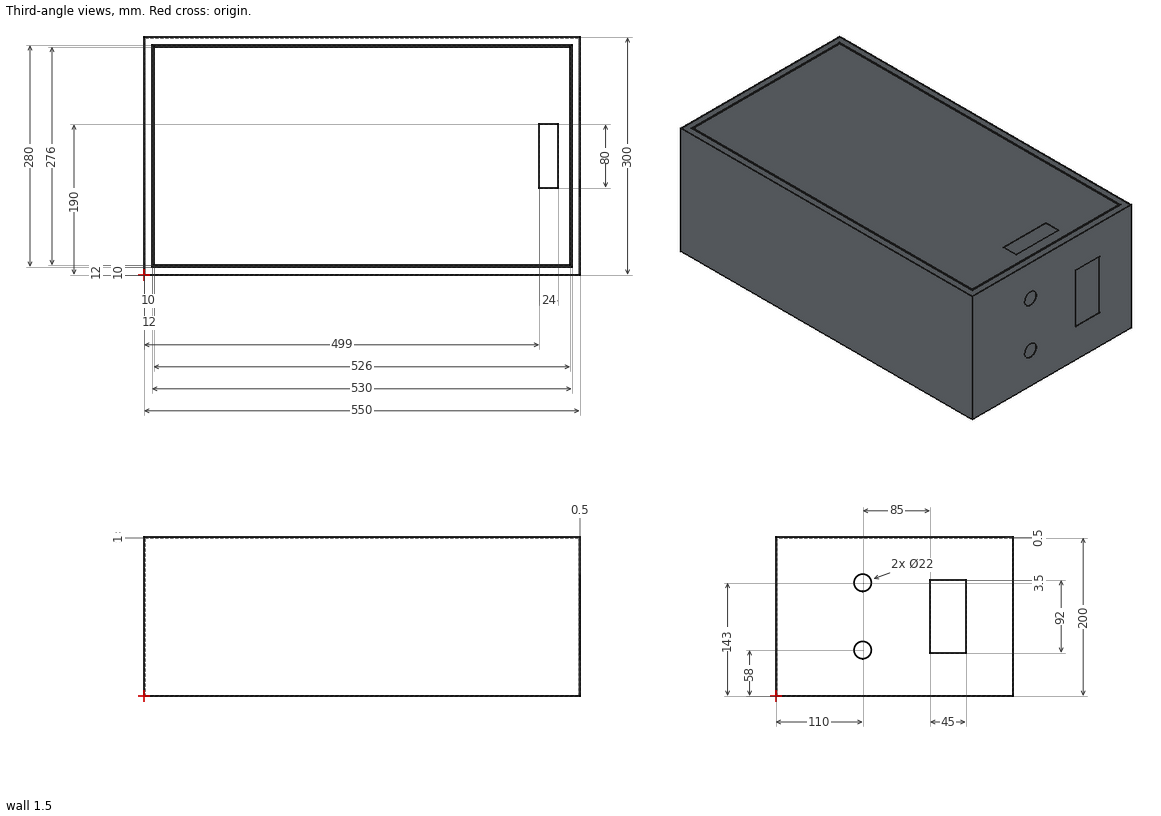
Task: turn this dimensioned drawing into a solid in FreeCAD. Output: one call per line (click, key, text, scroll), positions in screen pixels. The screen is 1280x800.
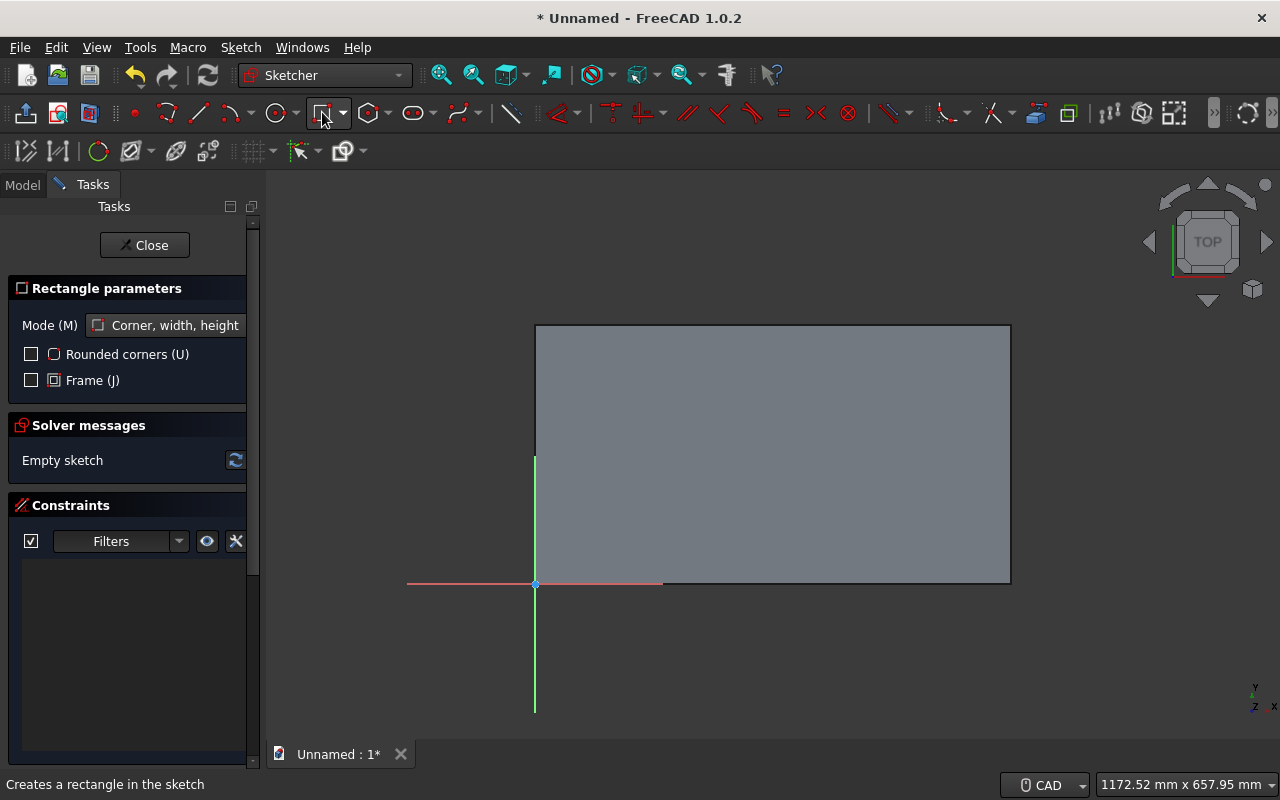
scroll(544, 333, up, 4)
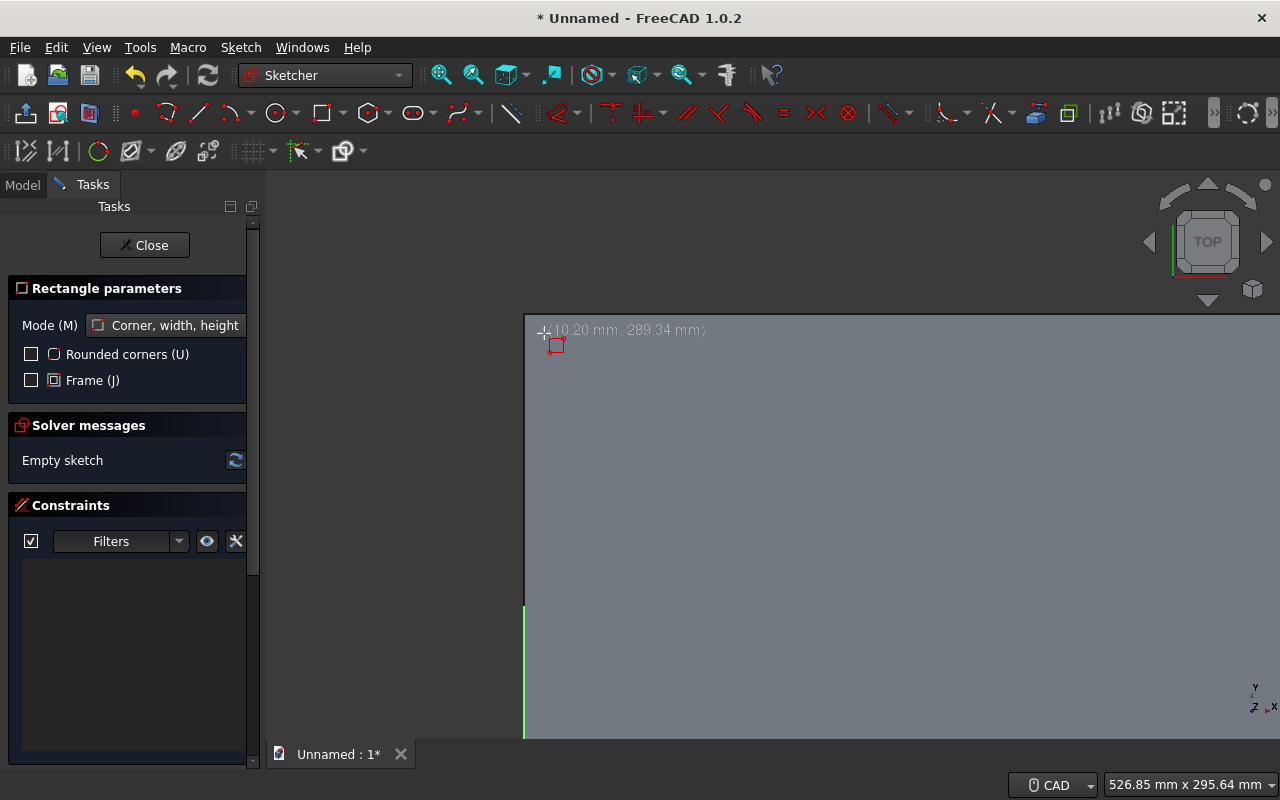
click(543, 334)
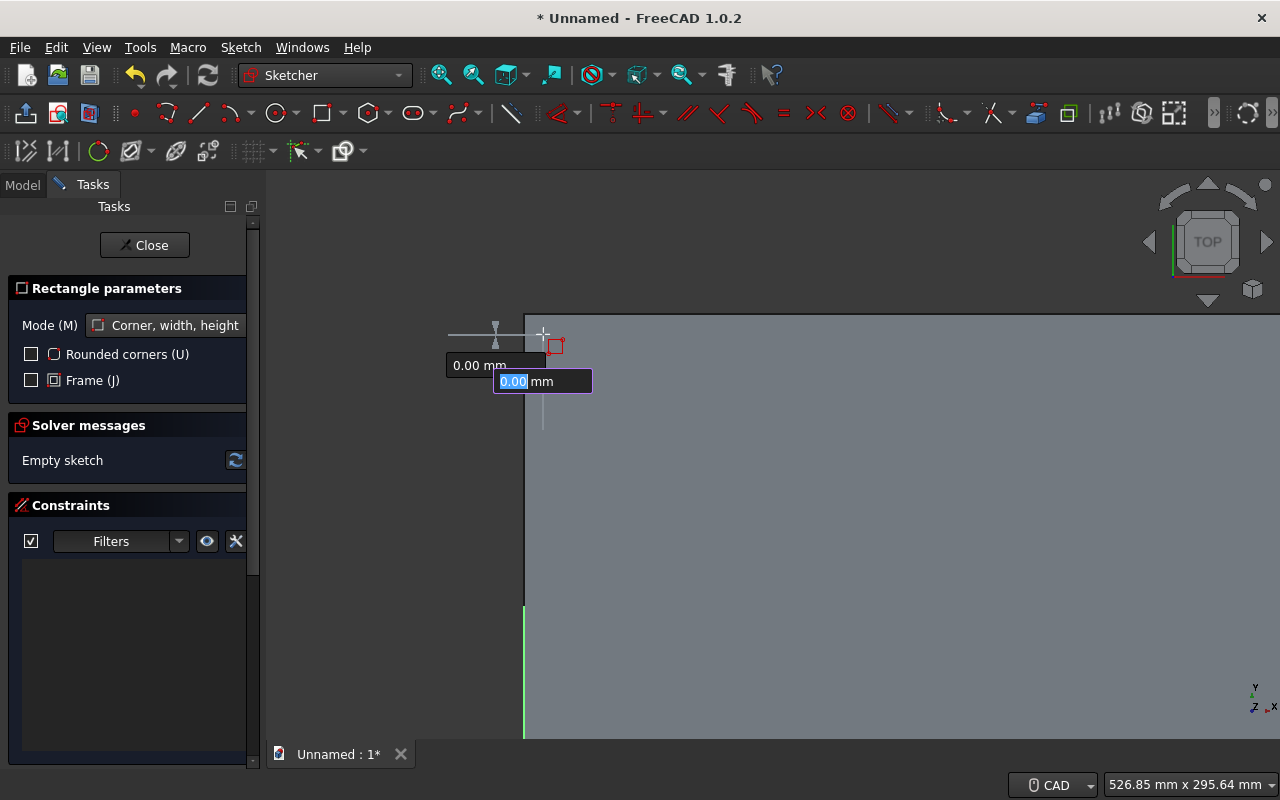
scroll(294, 262, down, 3)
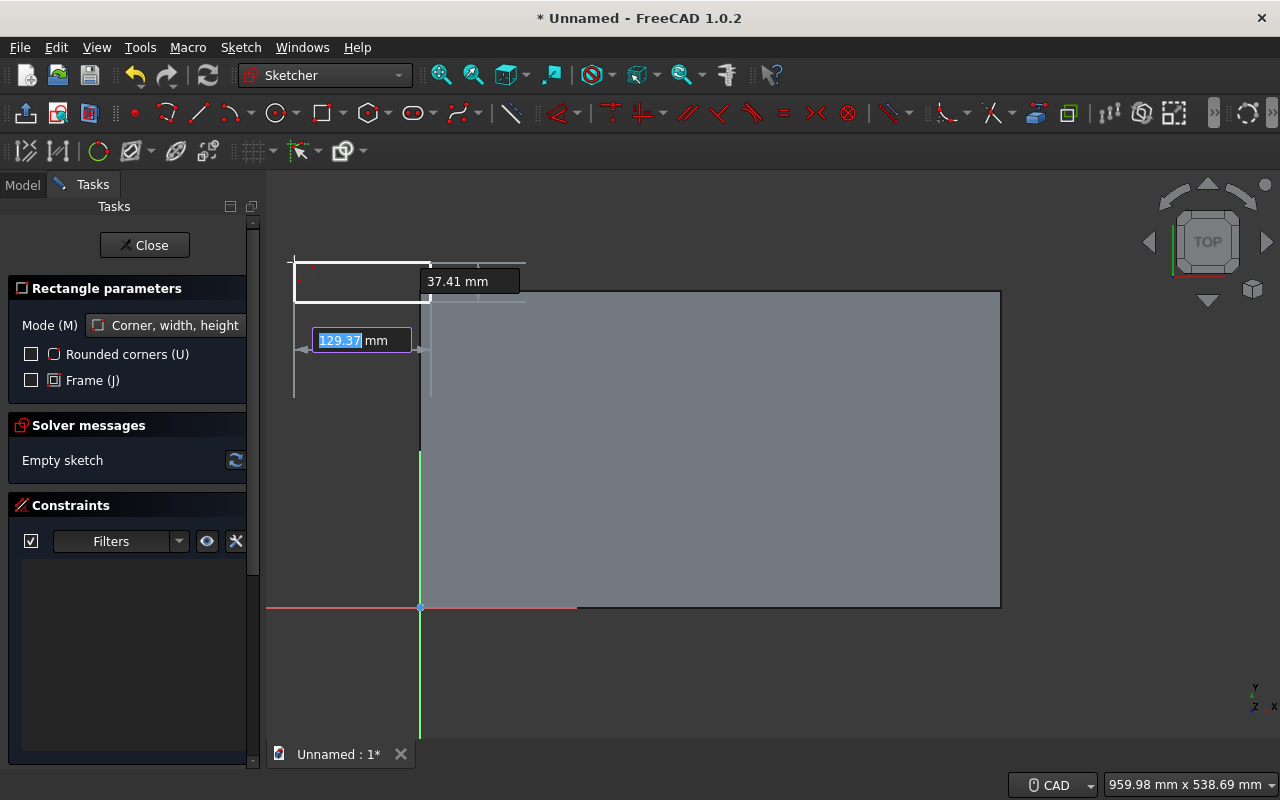
scroll(991, 597, up, 3)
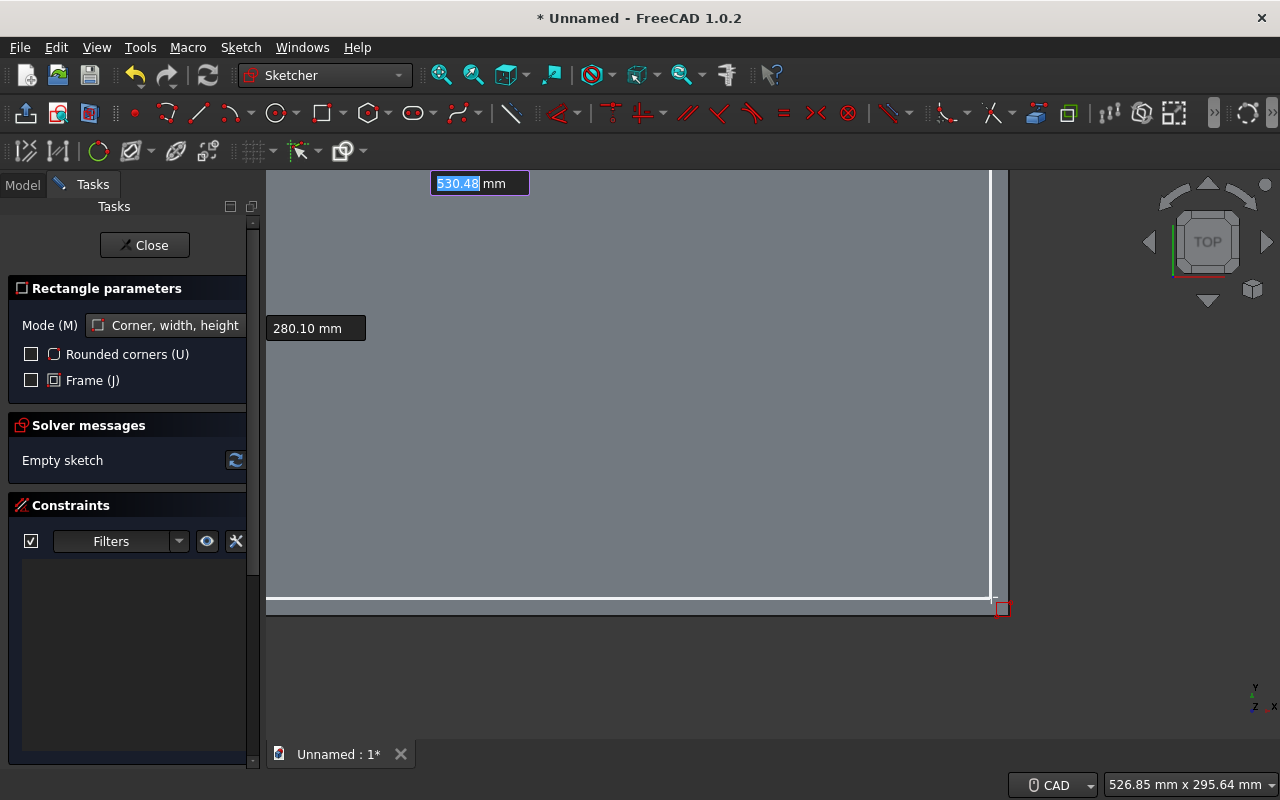
click(990, 597)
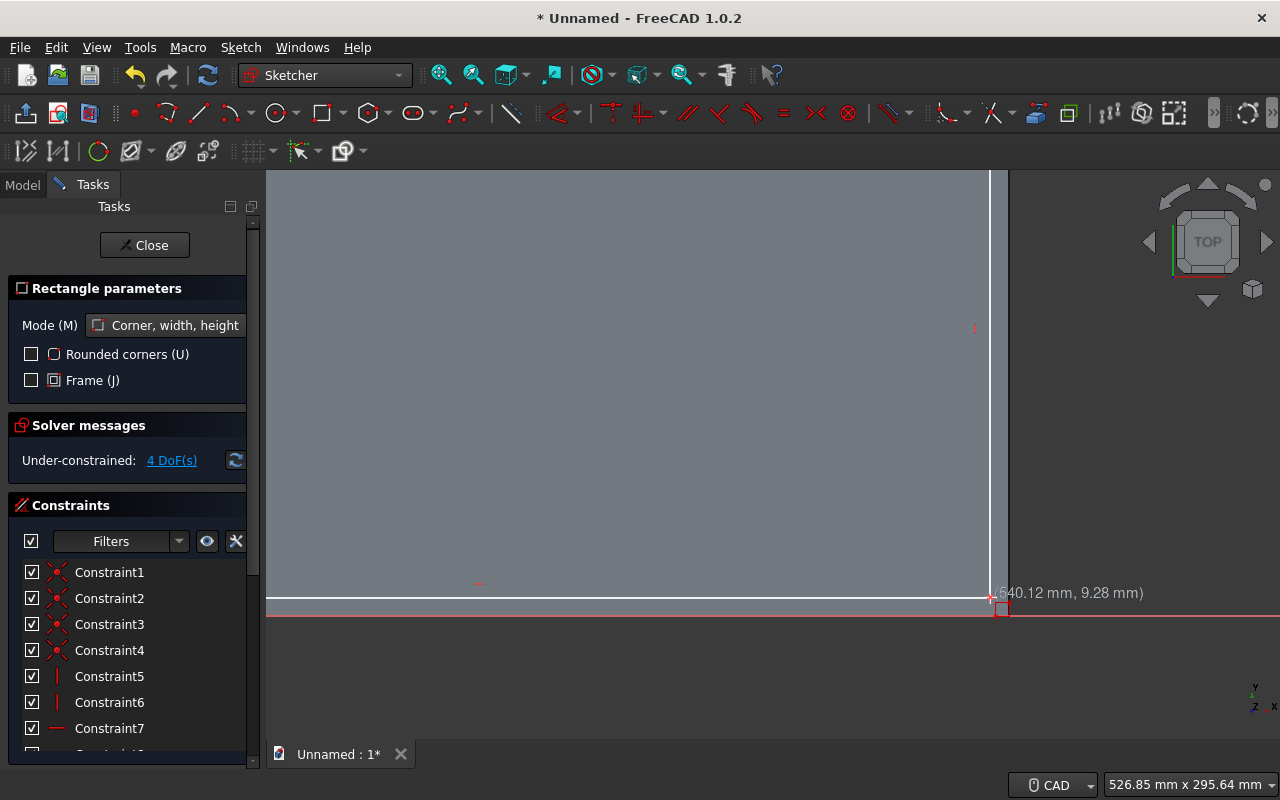
click(911, 250)
move(957, 404)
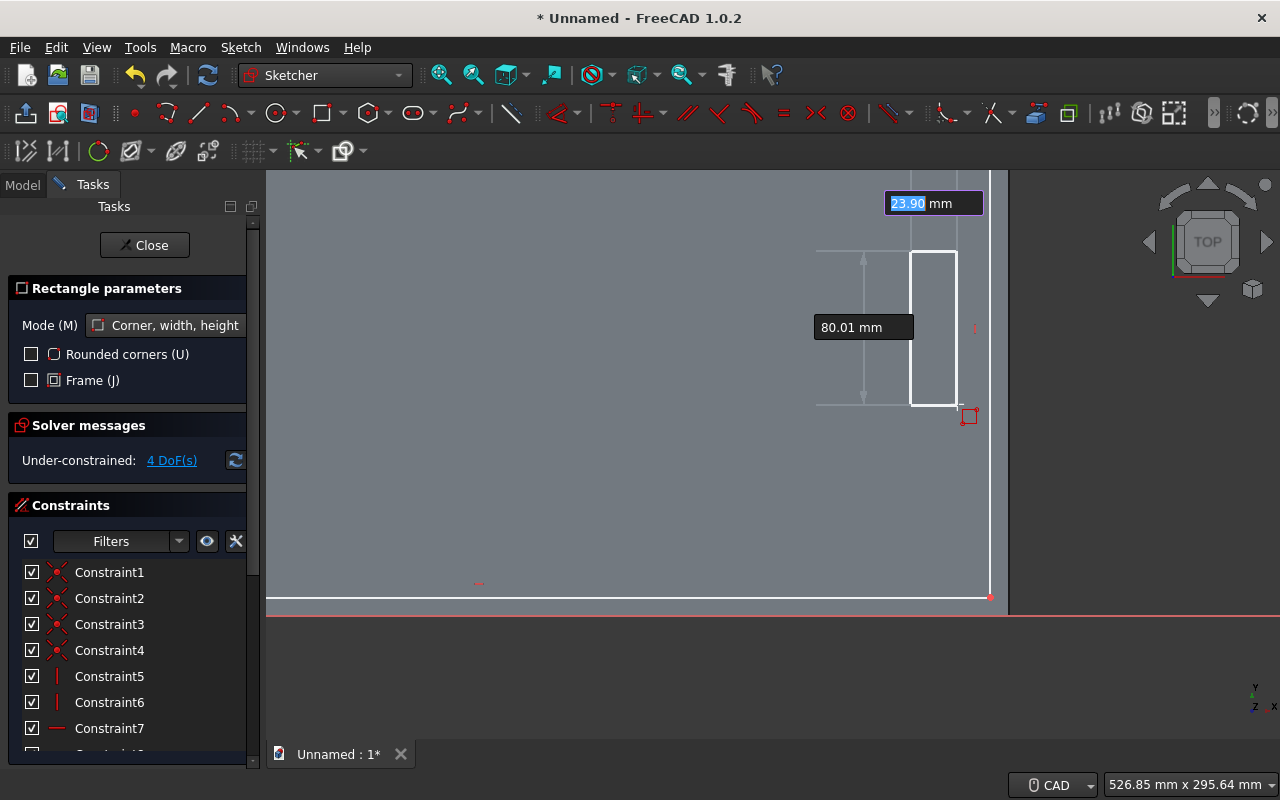
text(24)
key(Tab)
text(80)
key(Return)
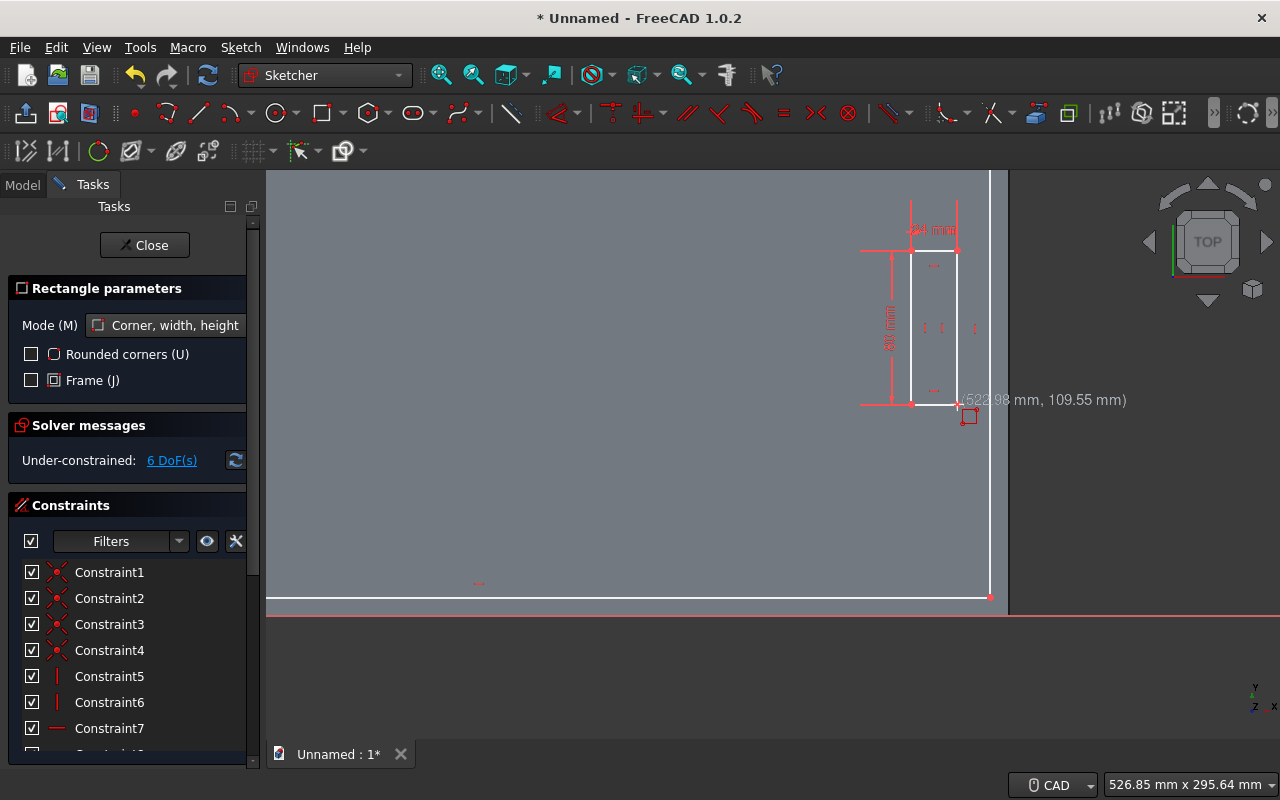
scroll(990, 598, down, 3)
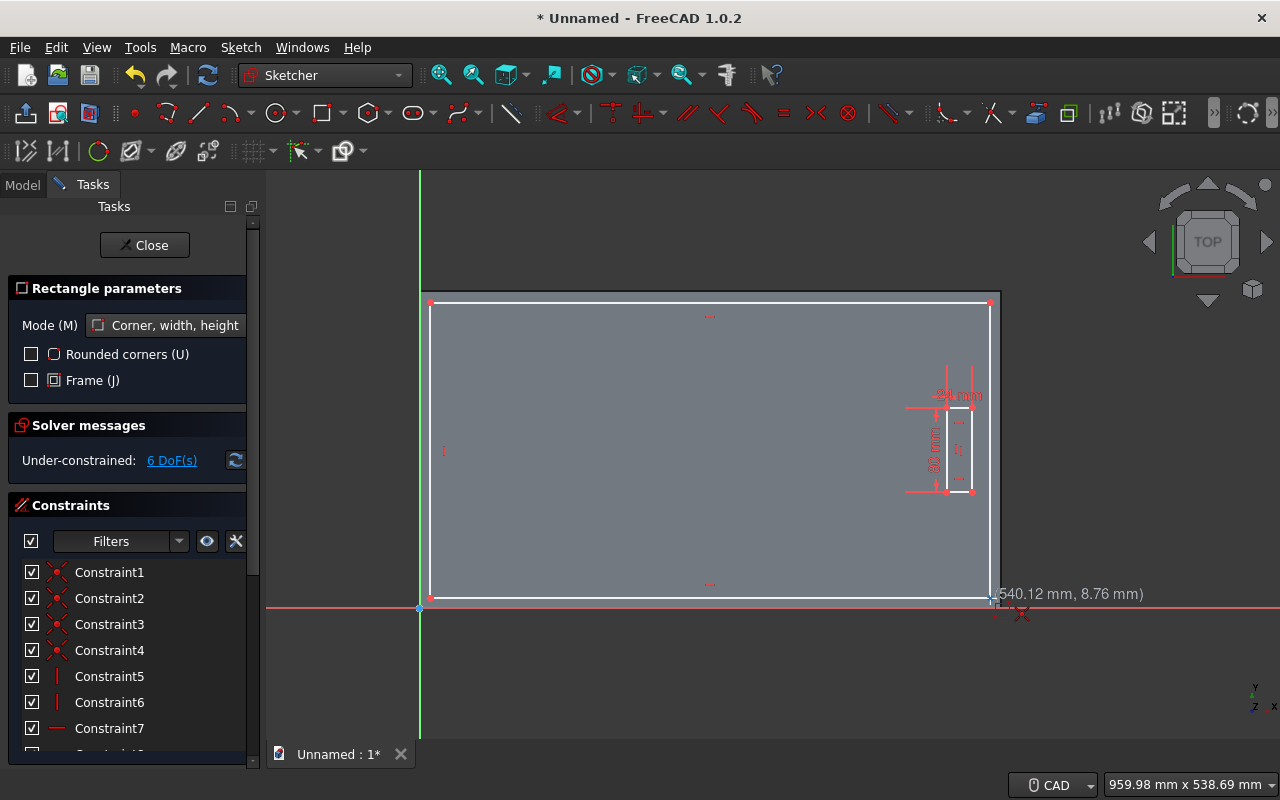
scroll(432, 304, up, 11)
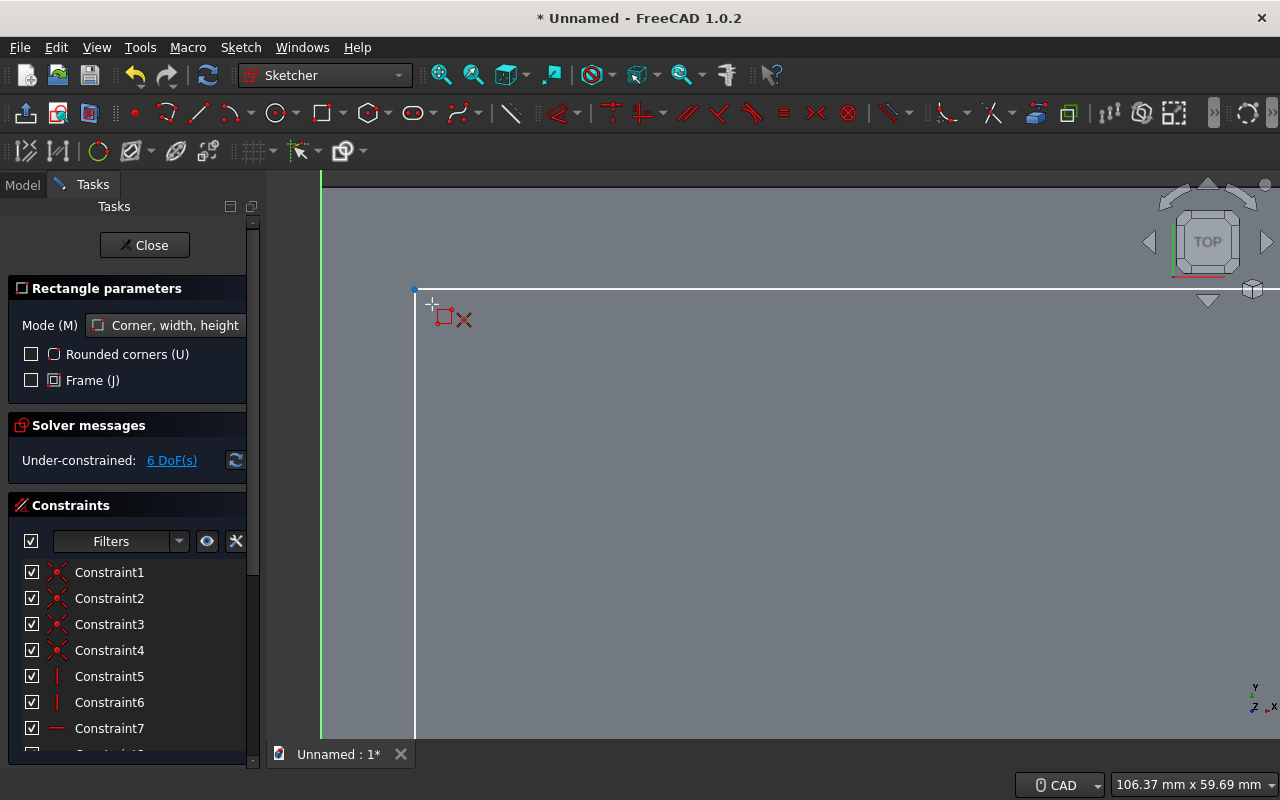
click(435, 301)